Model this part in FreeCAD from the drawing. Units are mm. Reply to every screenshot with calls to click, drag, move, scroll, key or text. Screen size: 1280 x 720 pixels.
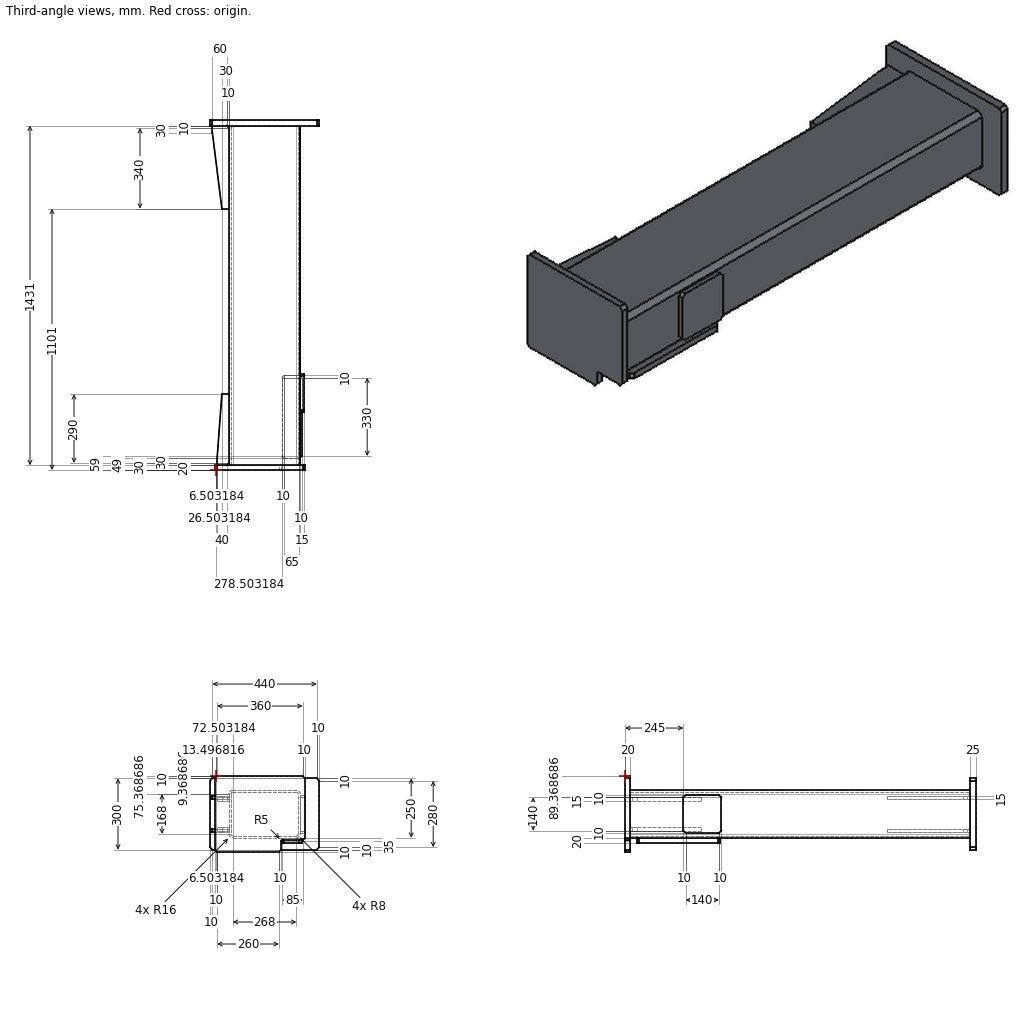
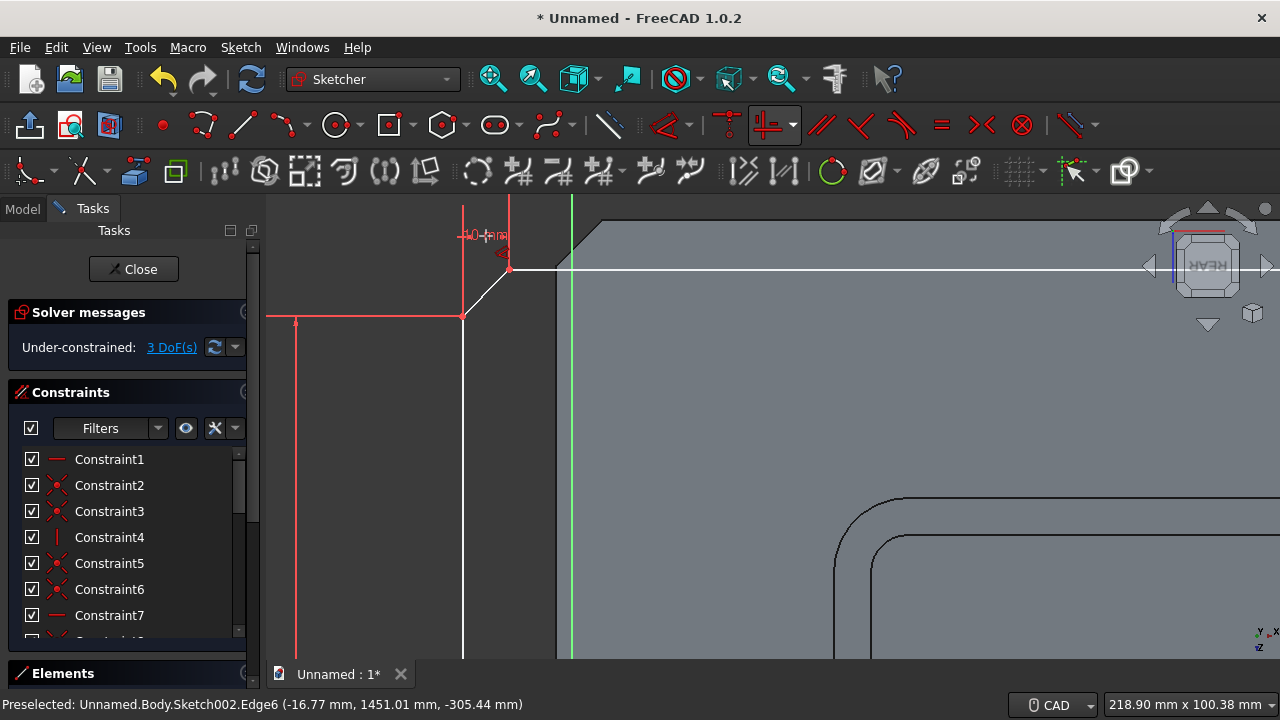
click(495, 284)
click(429, 293)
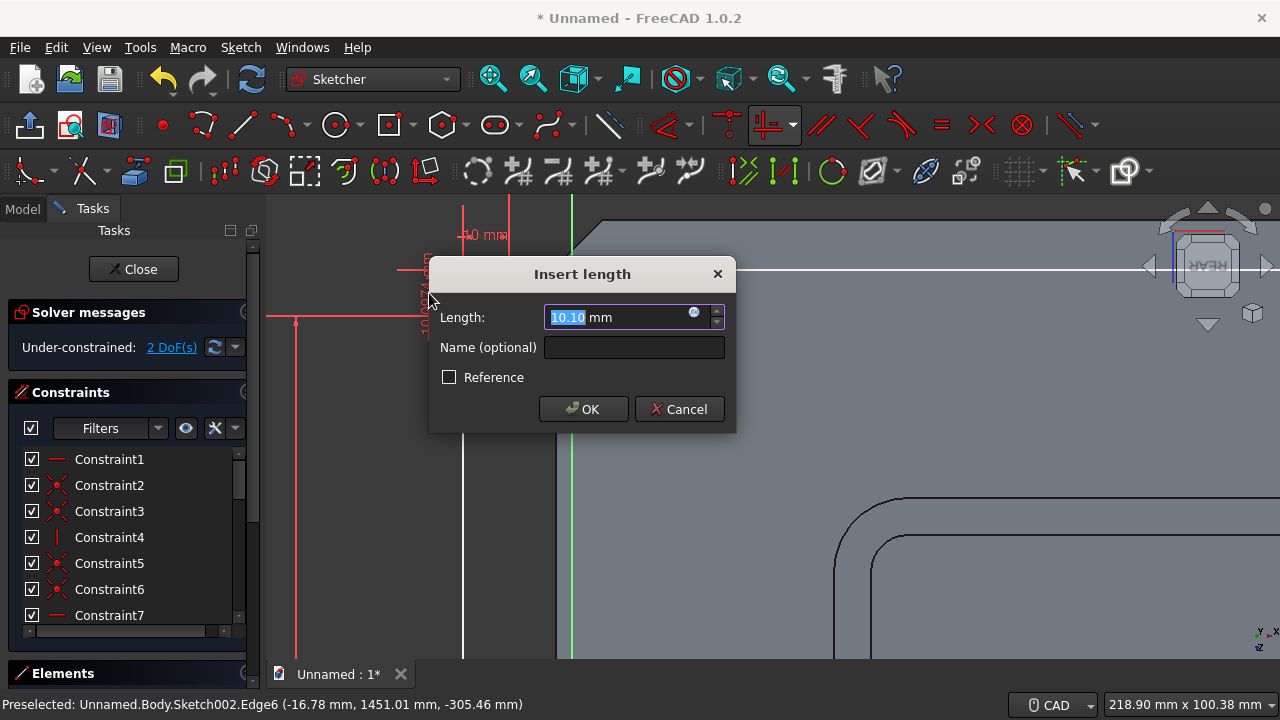
text(10)
key(Return)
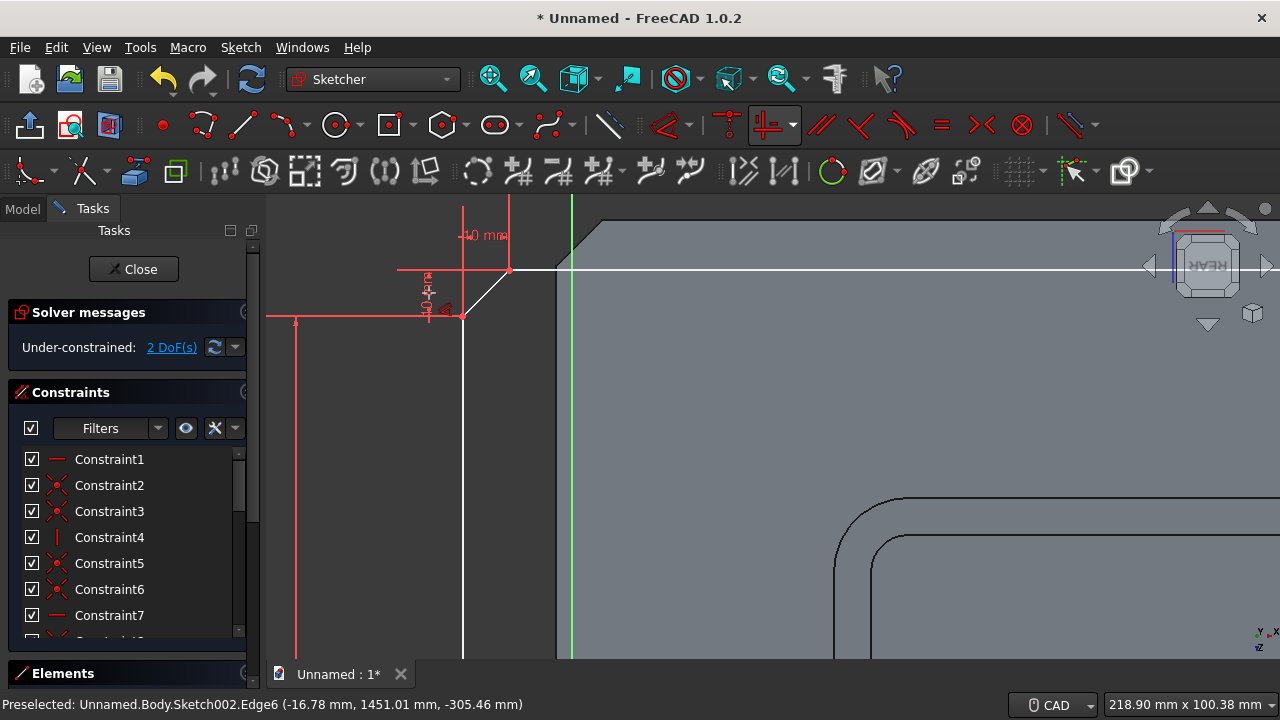
scroll(496, 286, down, 8)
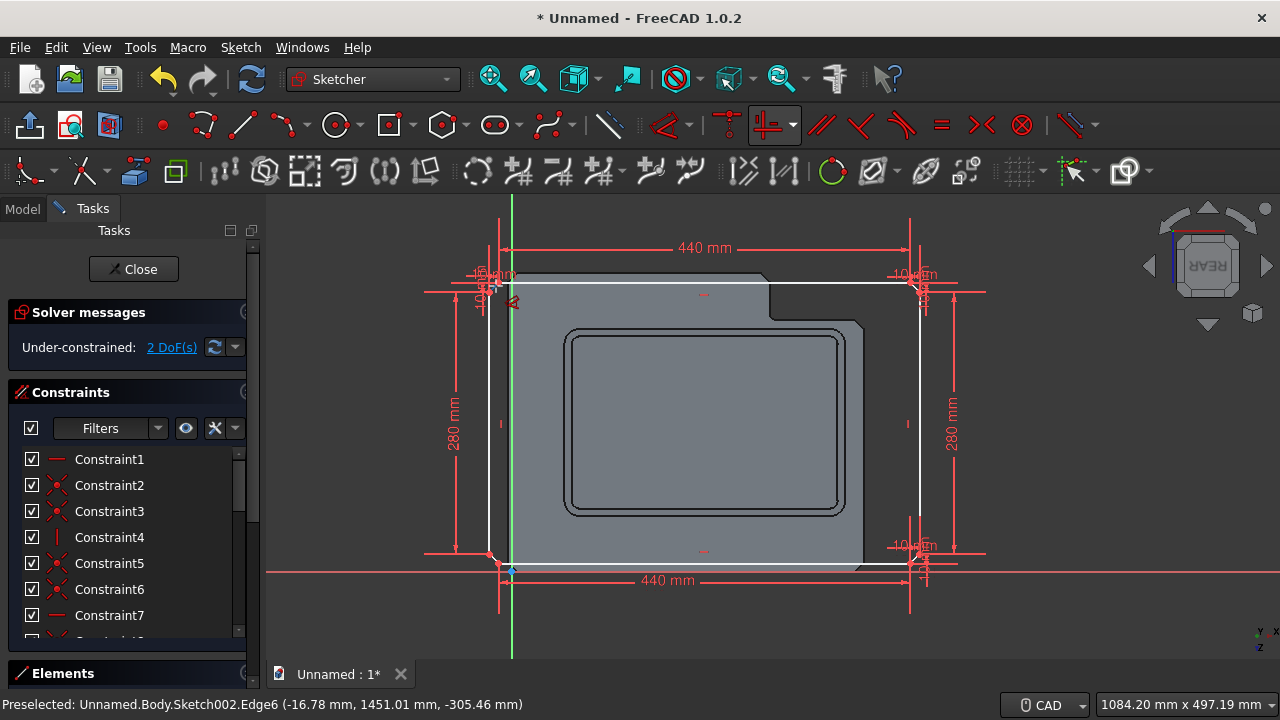
scroll(499, 564, up, 8)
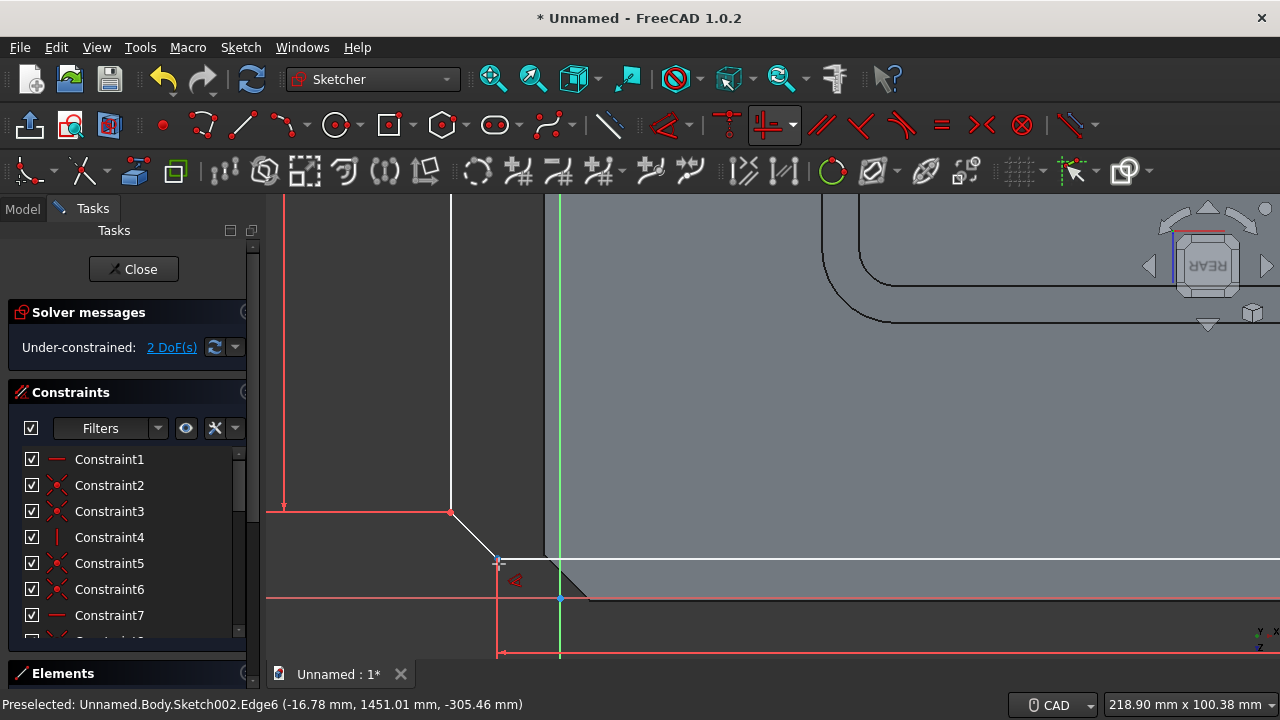
click(497, 559)
click(463, 578)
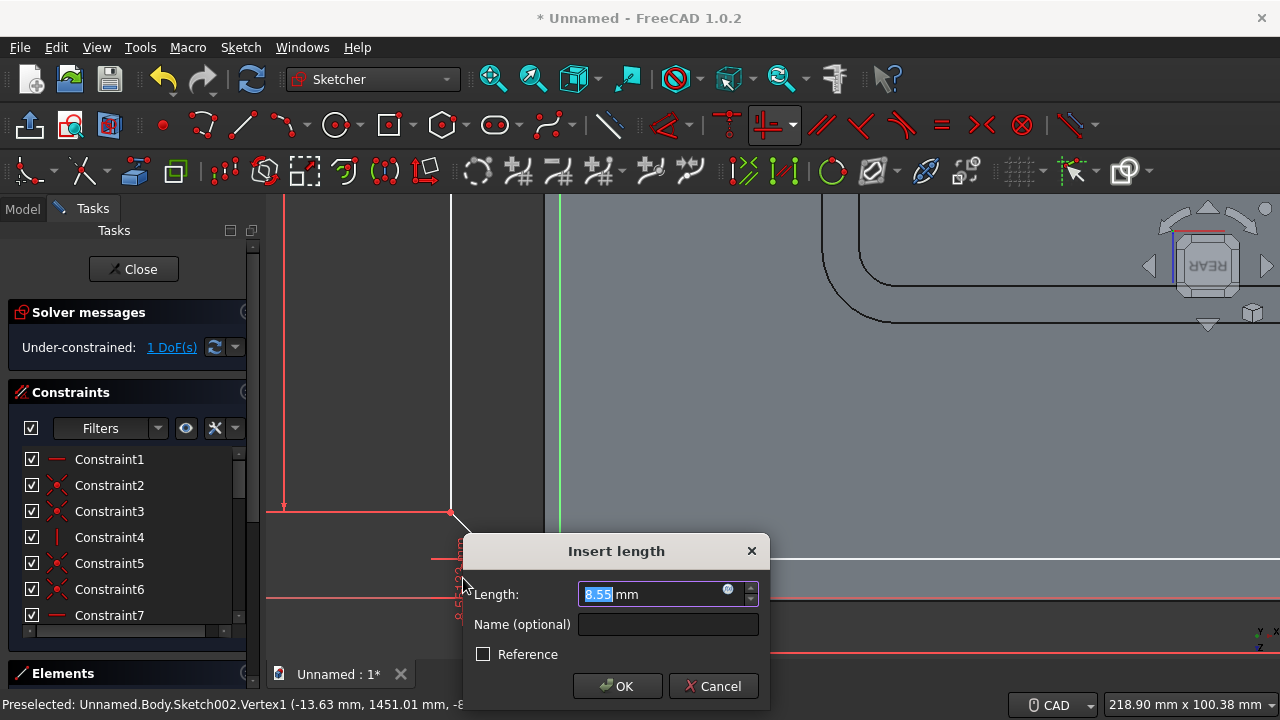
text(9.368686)
key(Return)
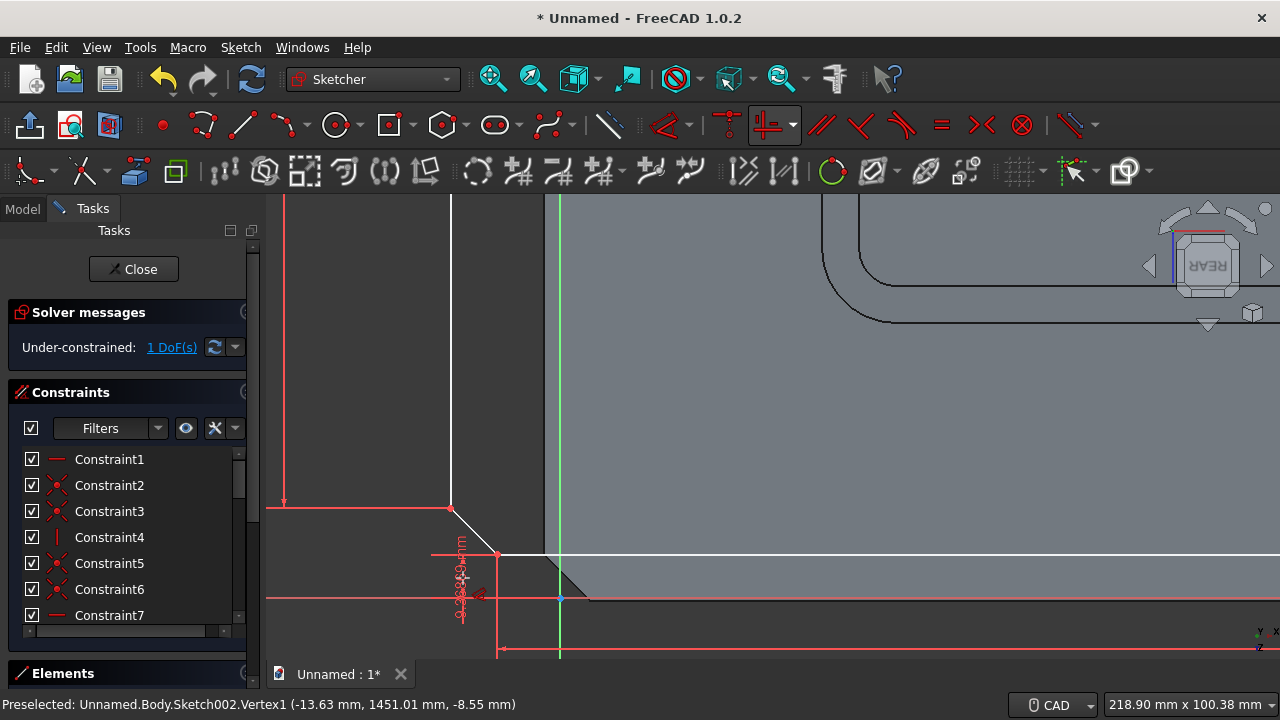
click(497, 555)
click(529, 521)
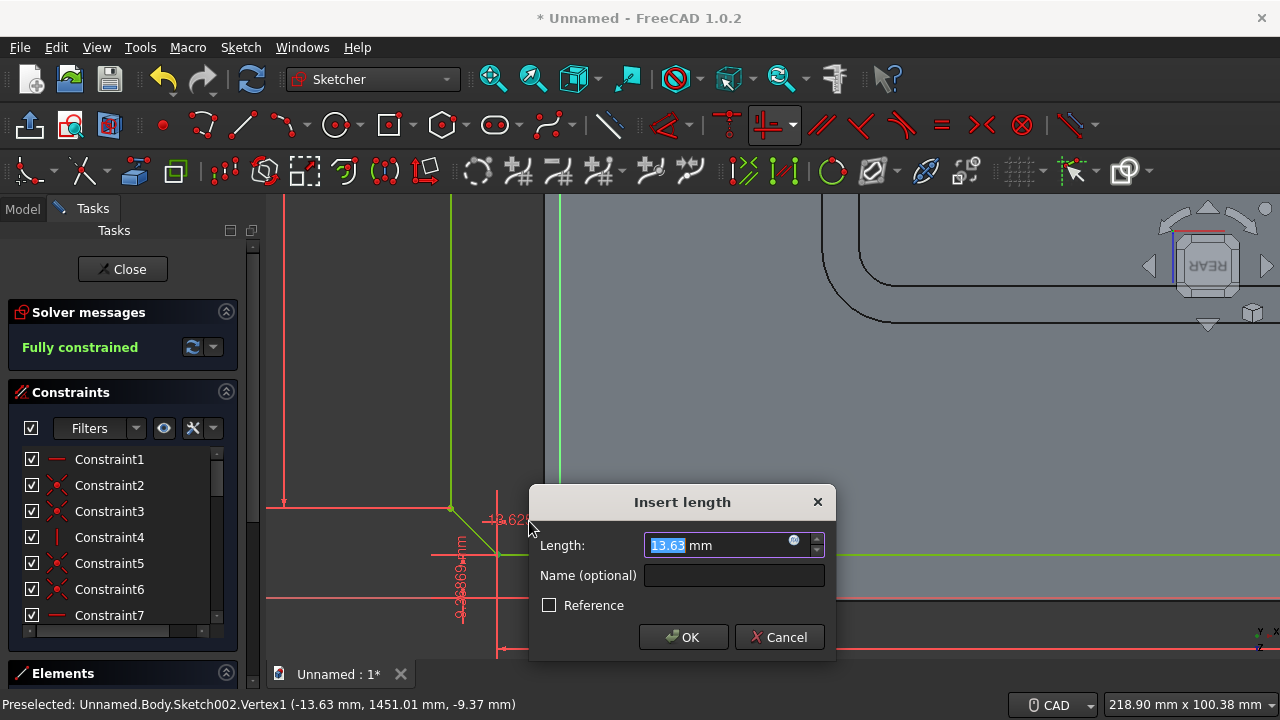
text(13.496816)
key(Return)
key(Escape)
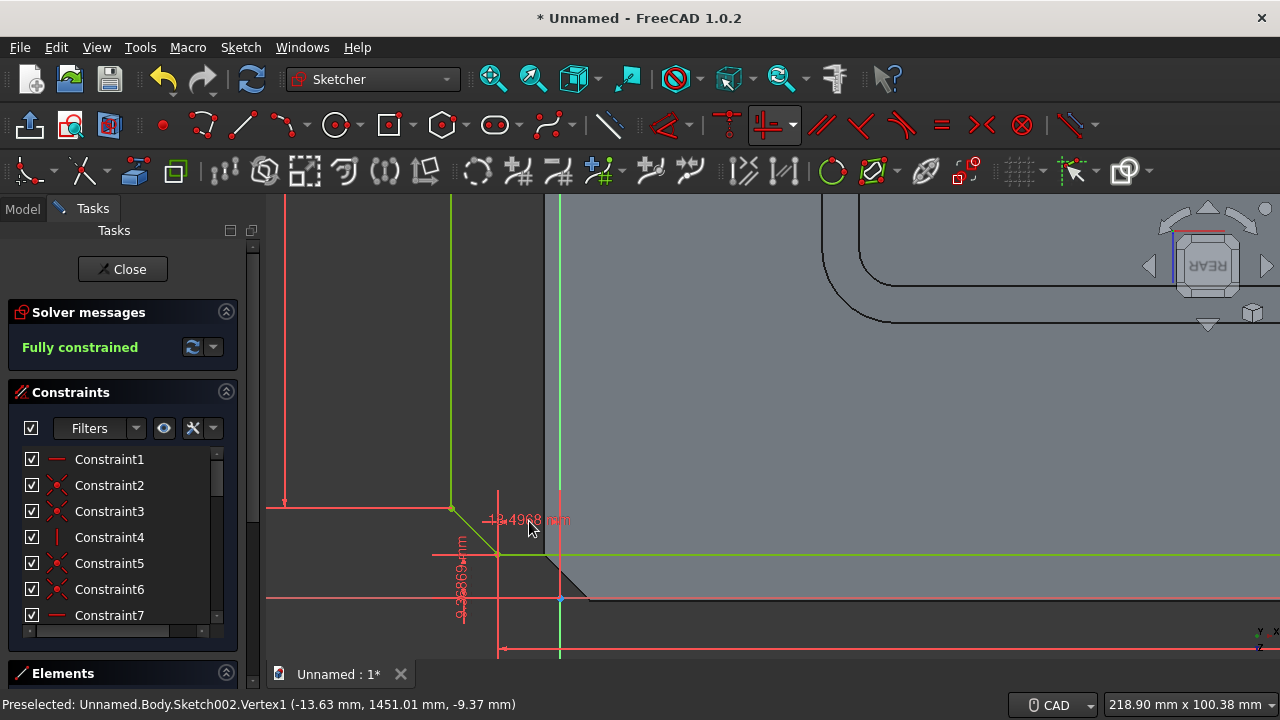
click(123, 269)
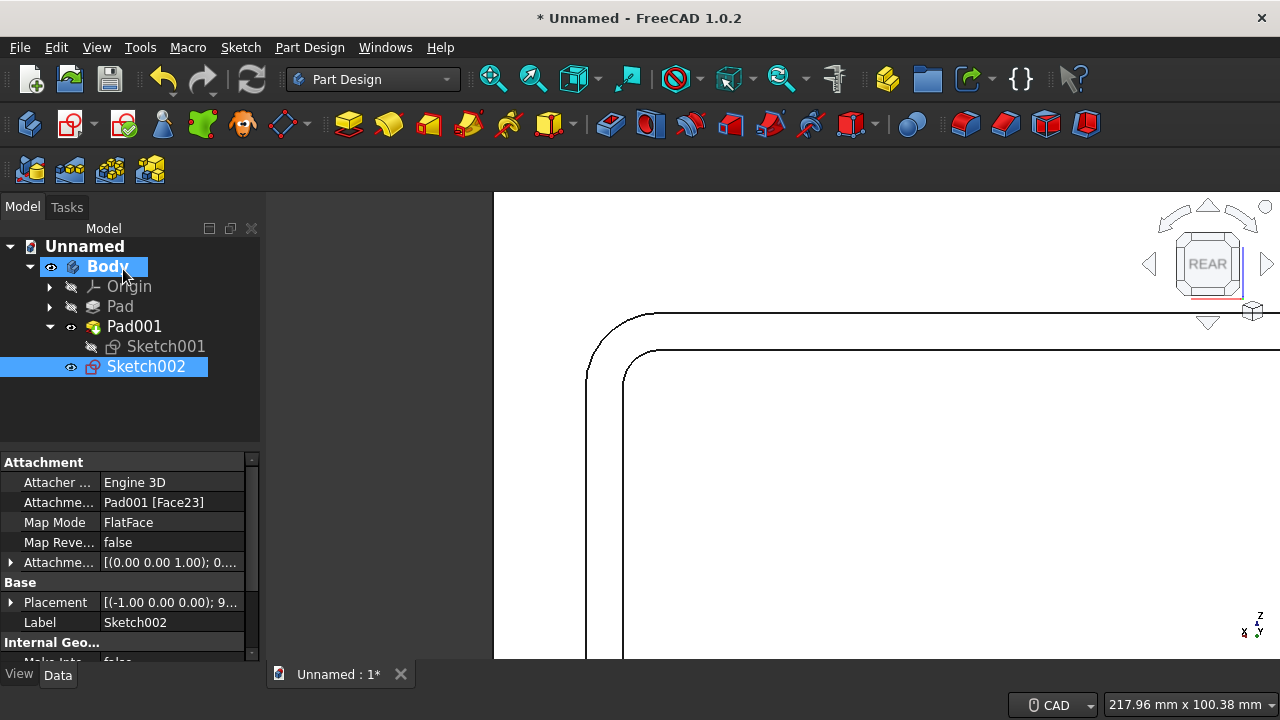
click(350, 124)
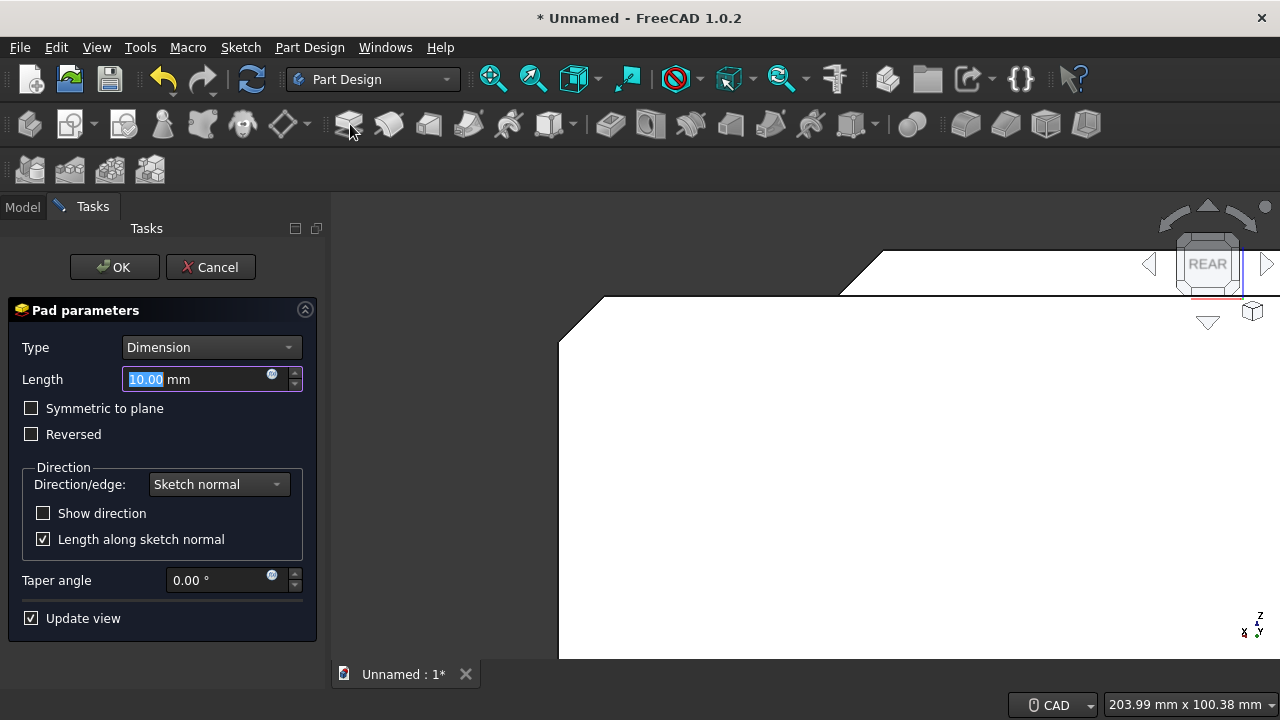
text(25)
key(Tab)